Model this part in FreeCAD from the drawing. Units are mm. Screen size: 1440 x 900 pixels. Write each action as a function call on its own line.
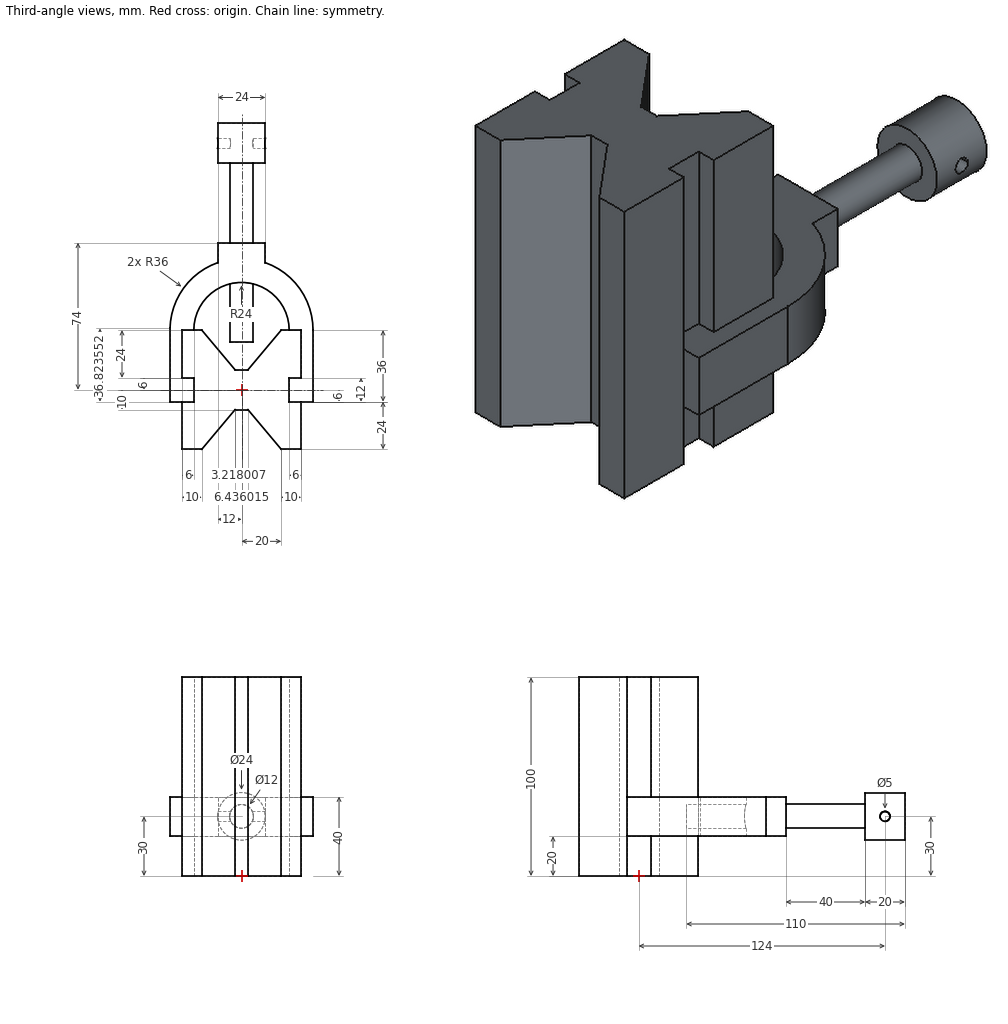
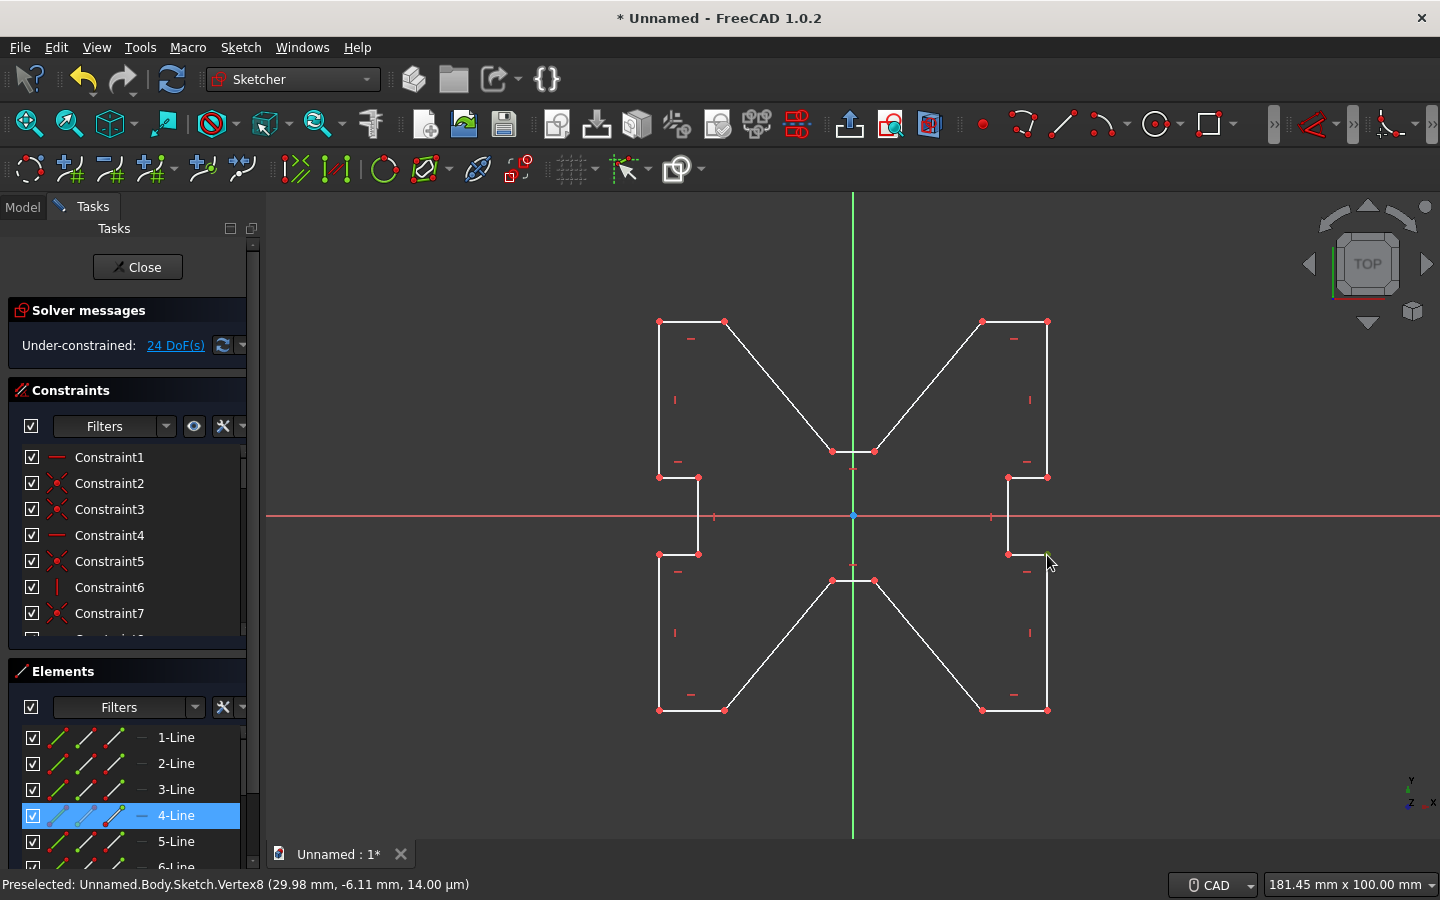
click(1047, 478)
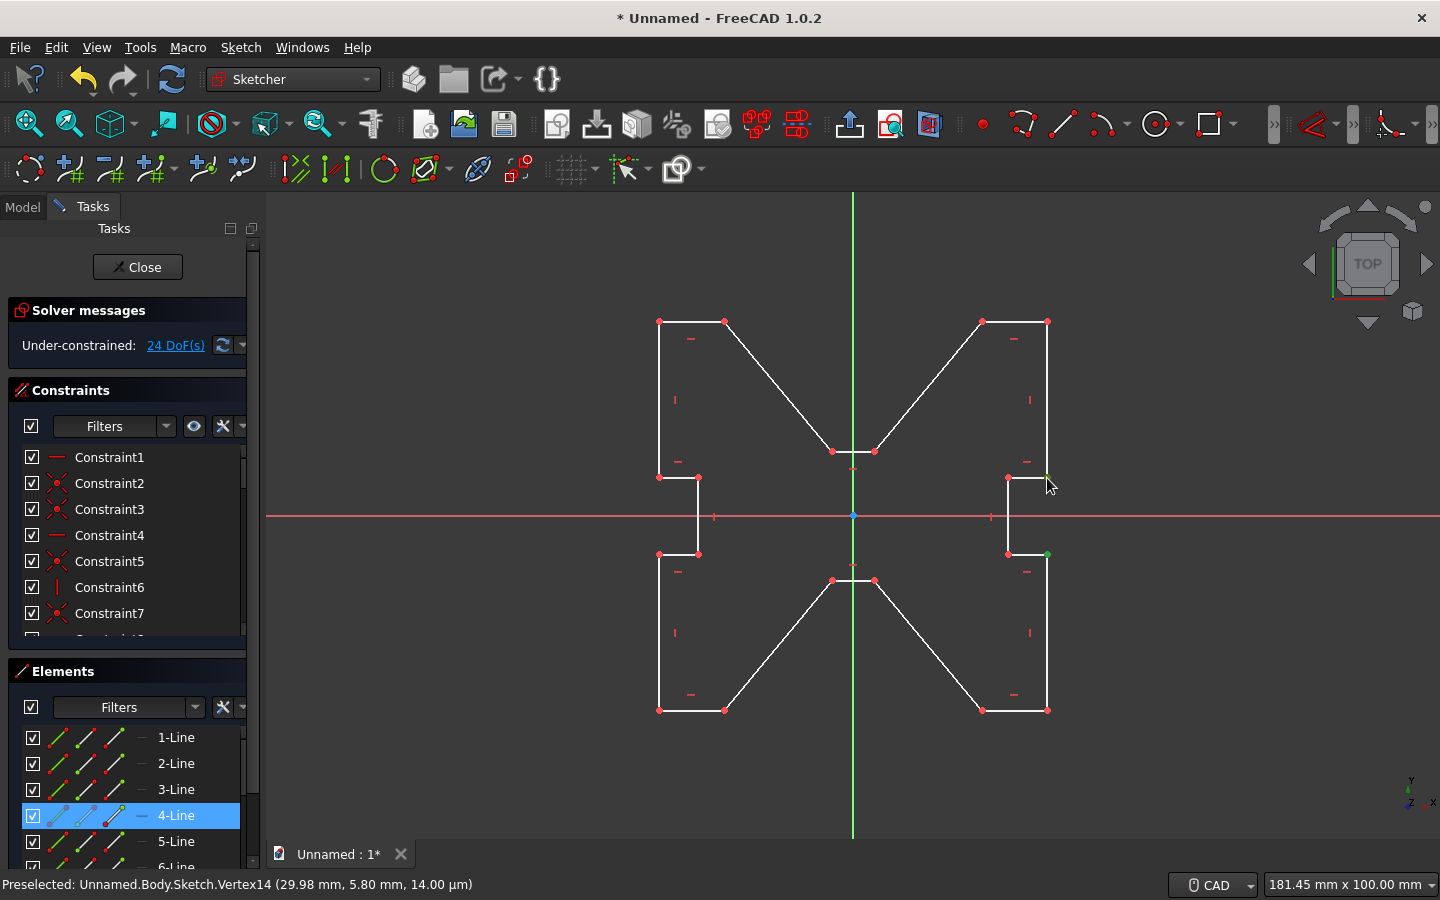
click(364, 516)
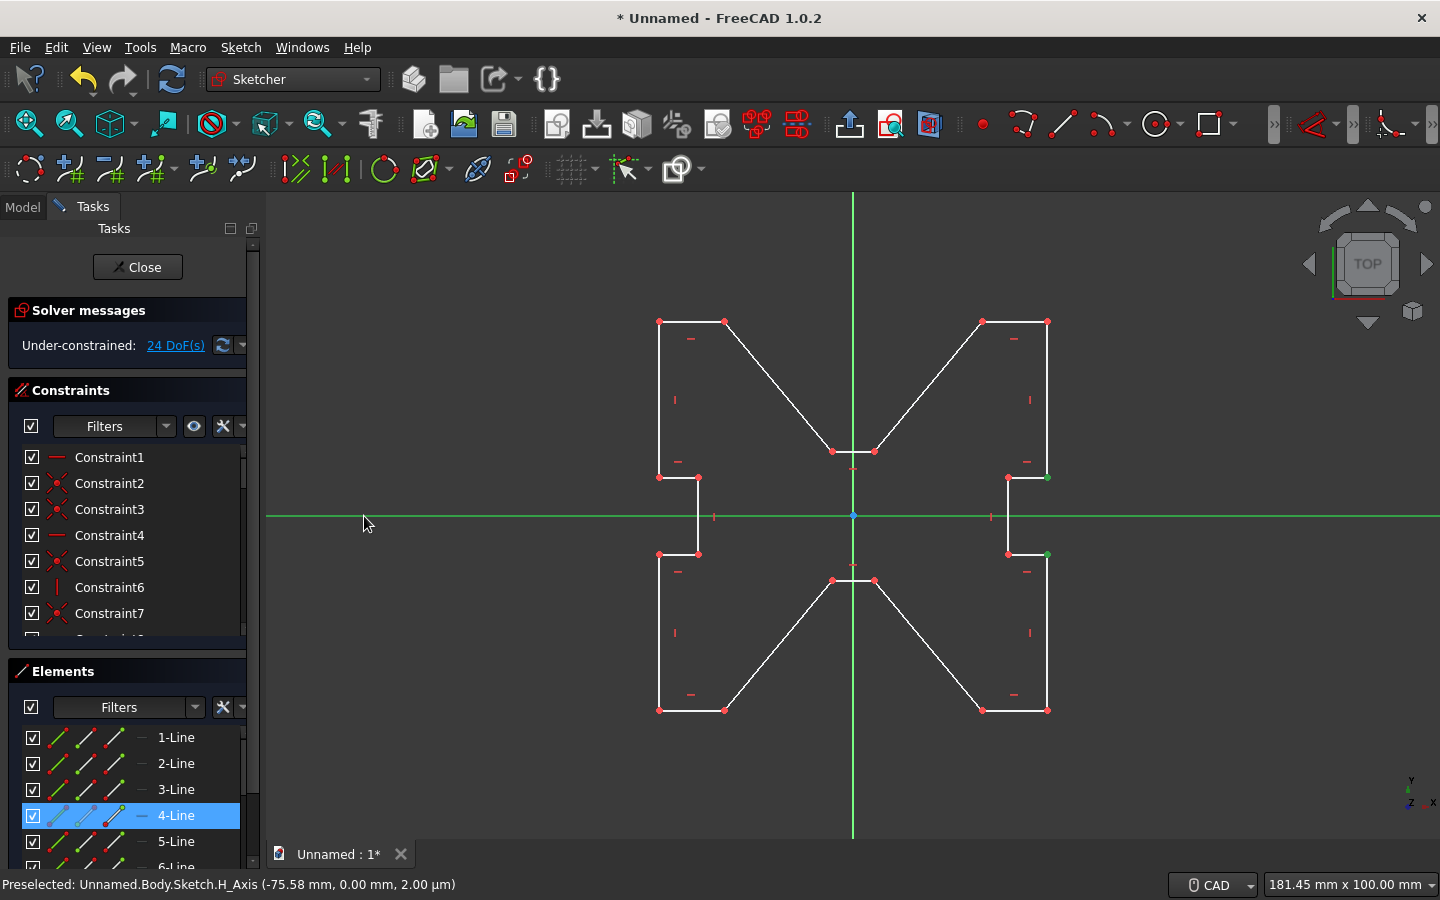
key(s)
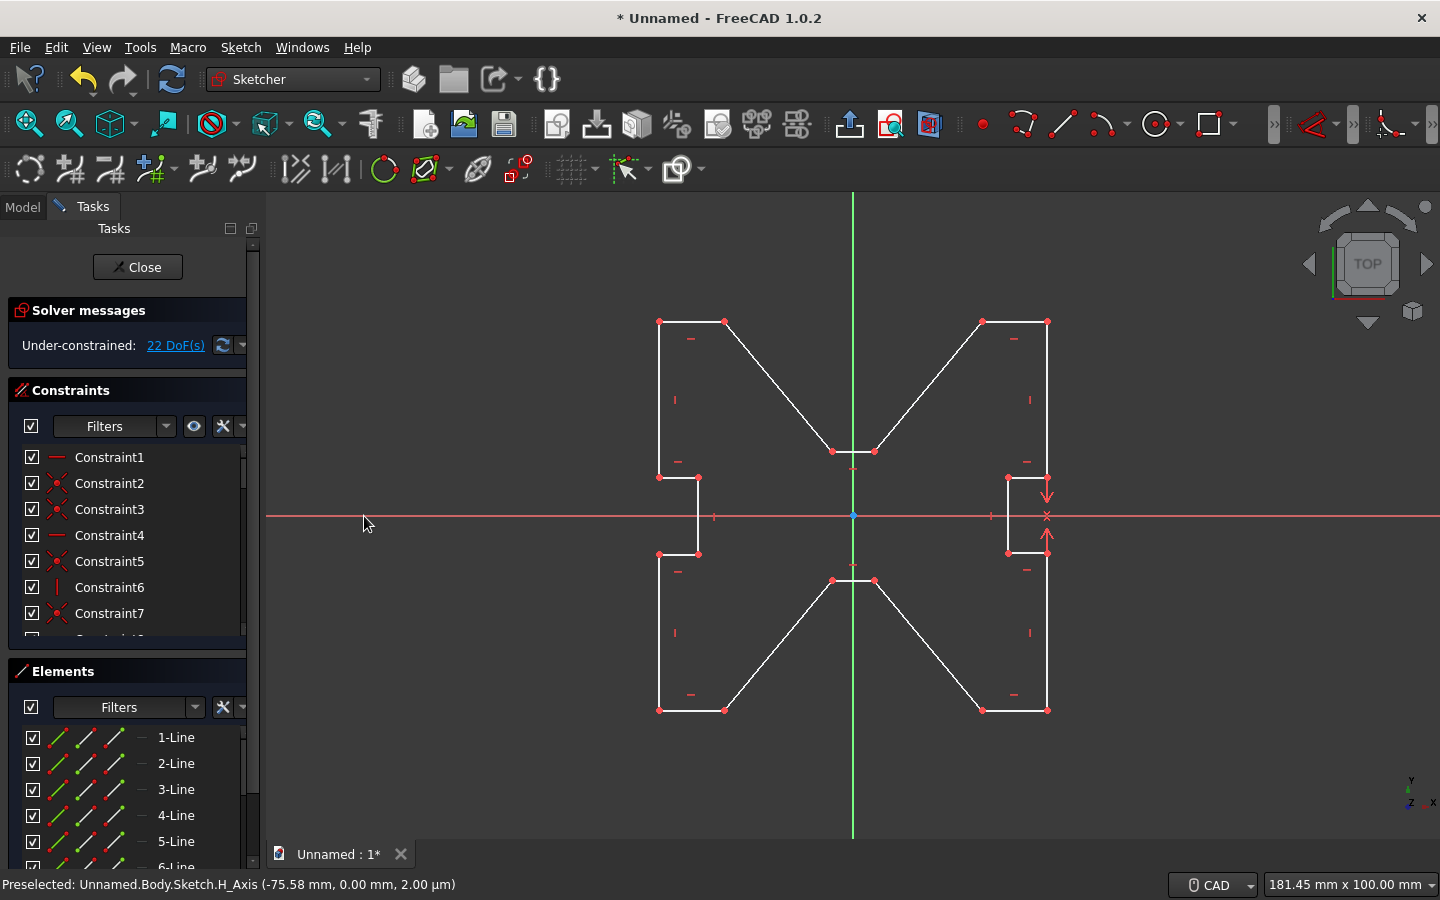
click(982, 711)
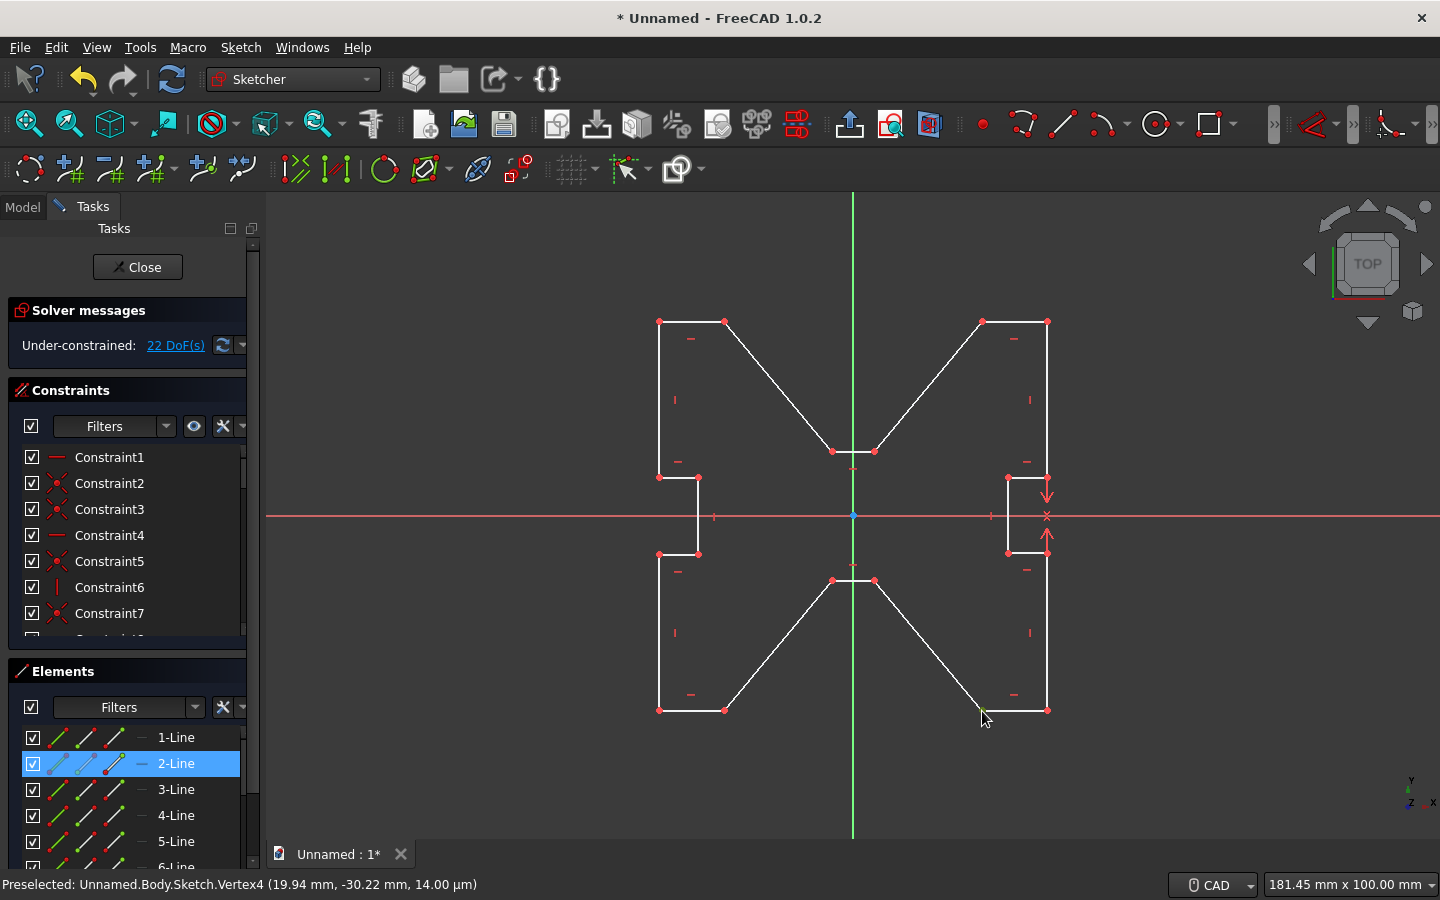
click(982, 322)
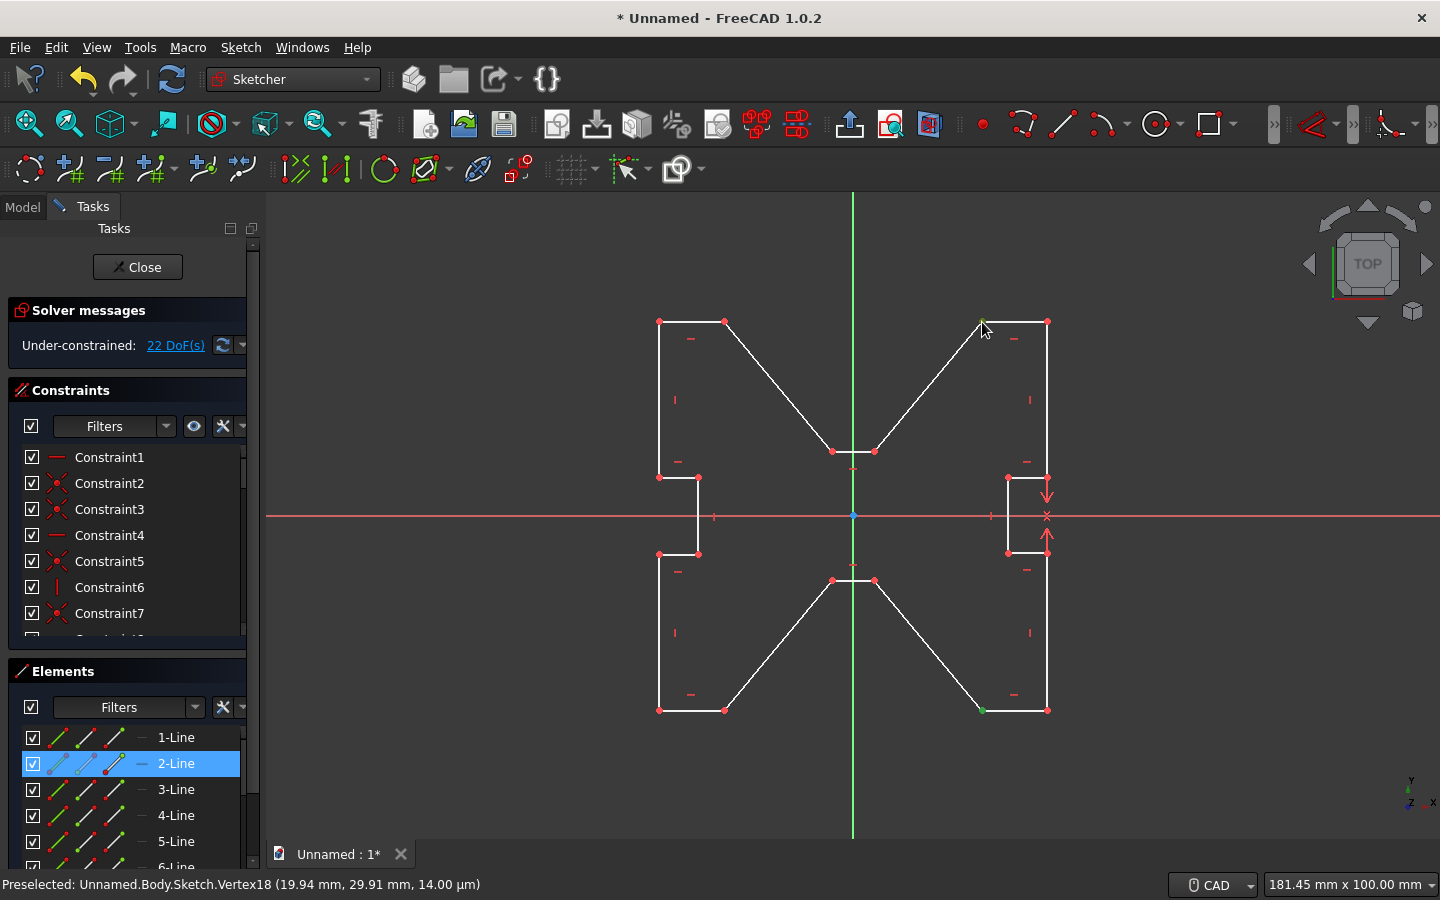
click(364, 516)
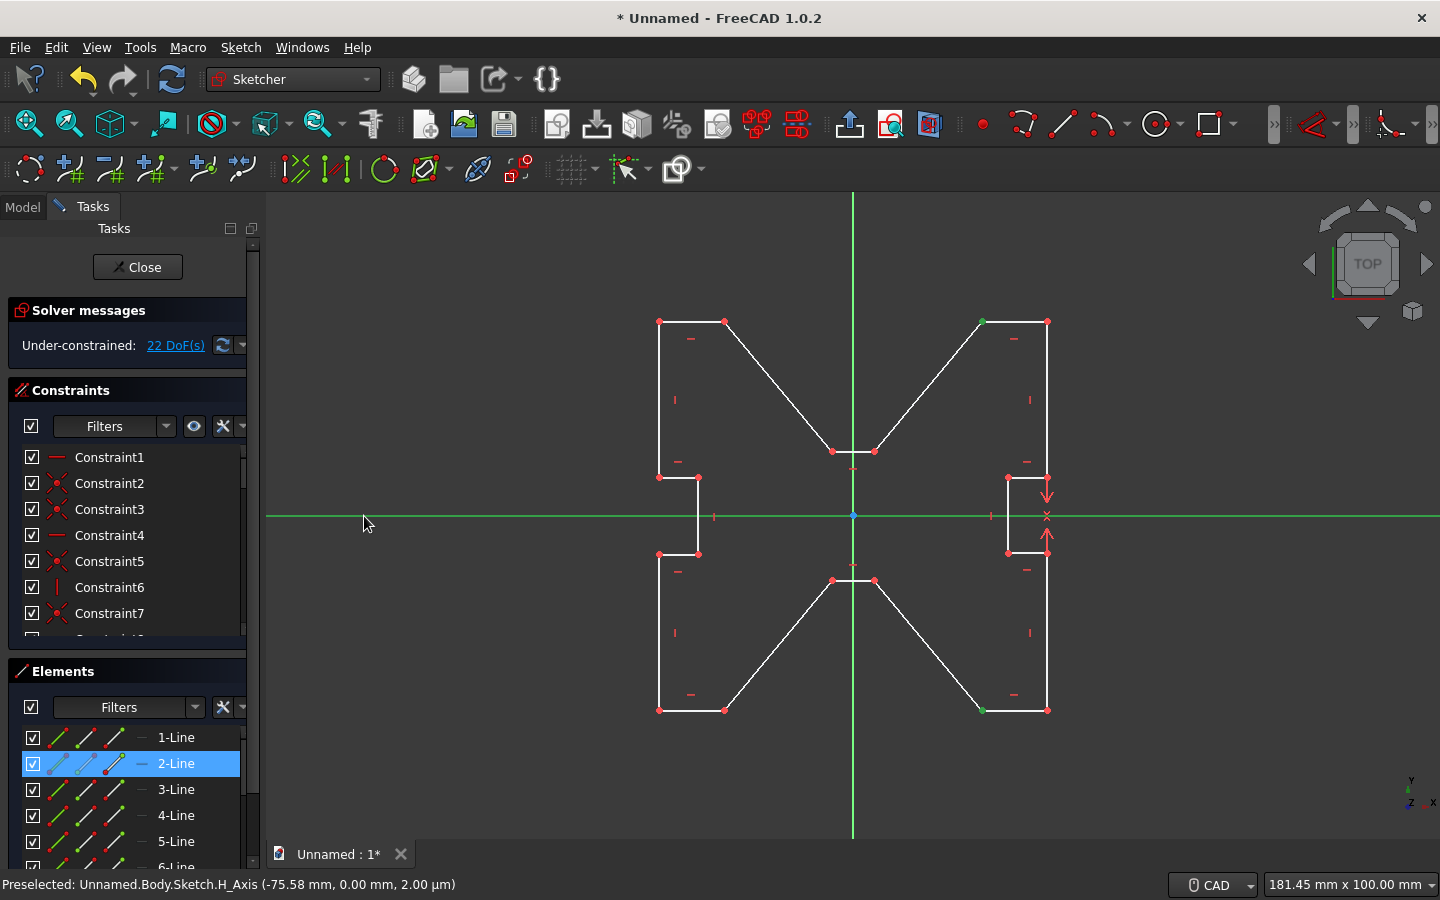
key(s)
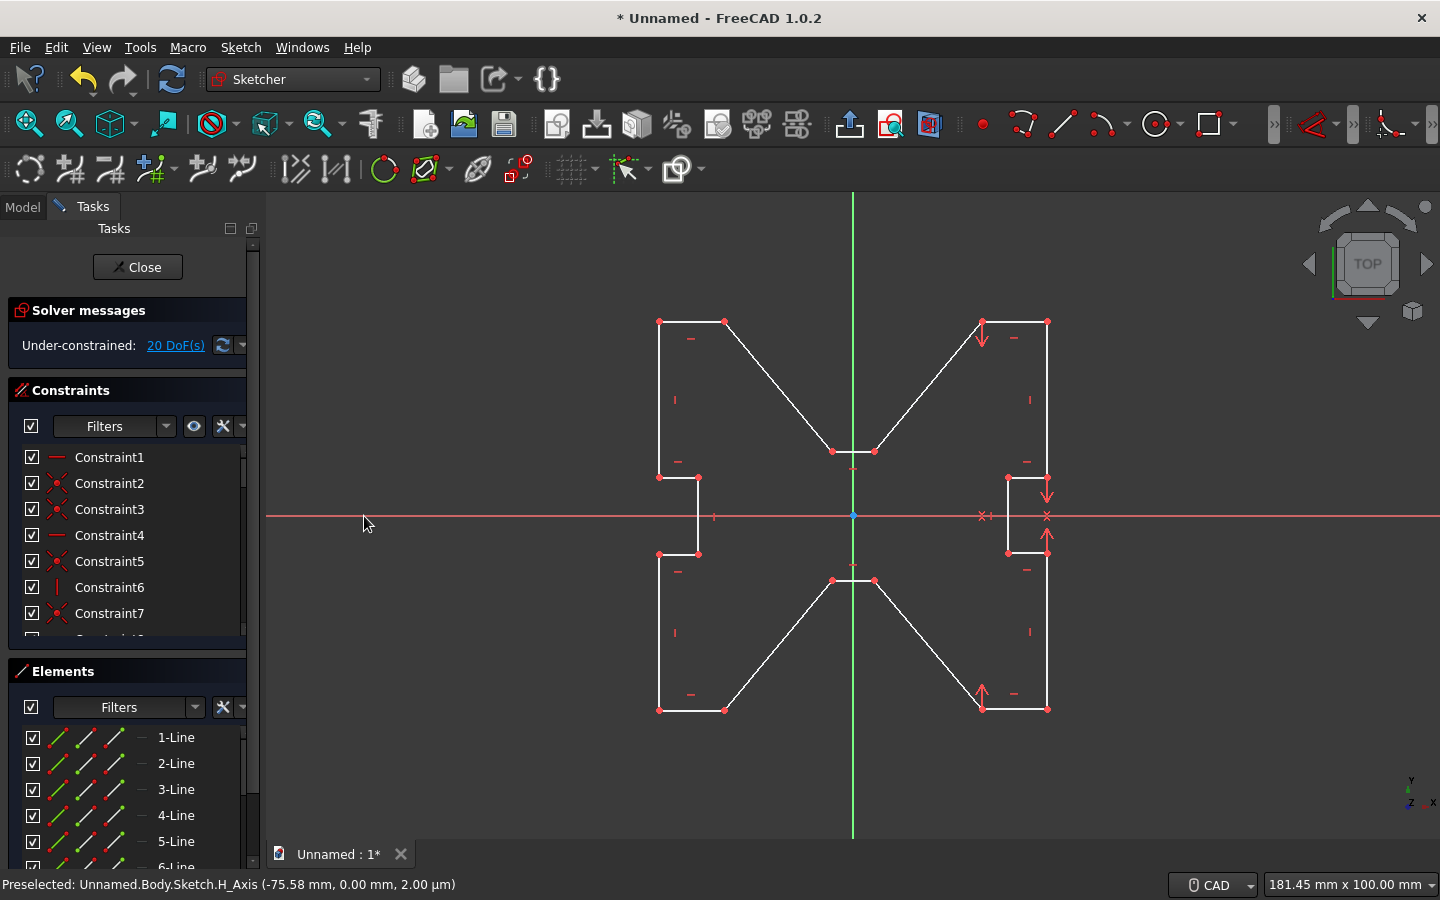
click(874, 581)